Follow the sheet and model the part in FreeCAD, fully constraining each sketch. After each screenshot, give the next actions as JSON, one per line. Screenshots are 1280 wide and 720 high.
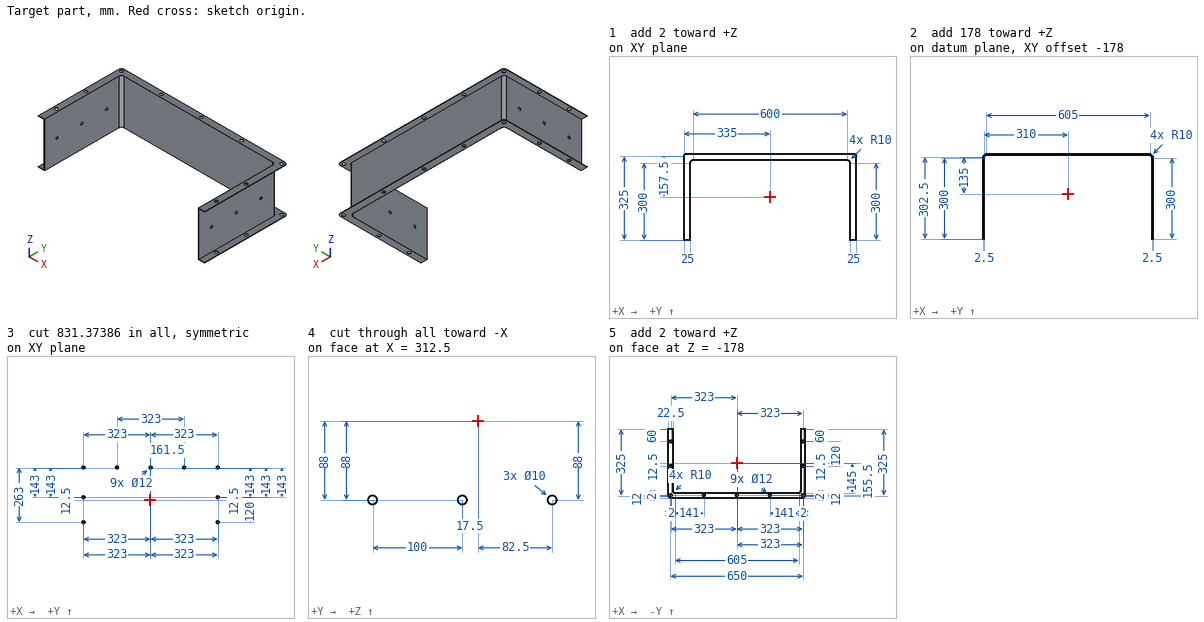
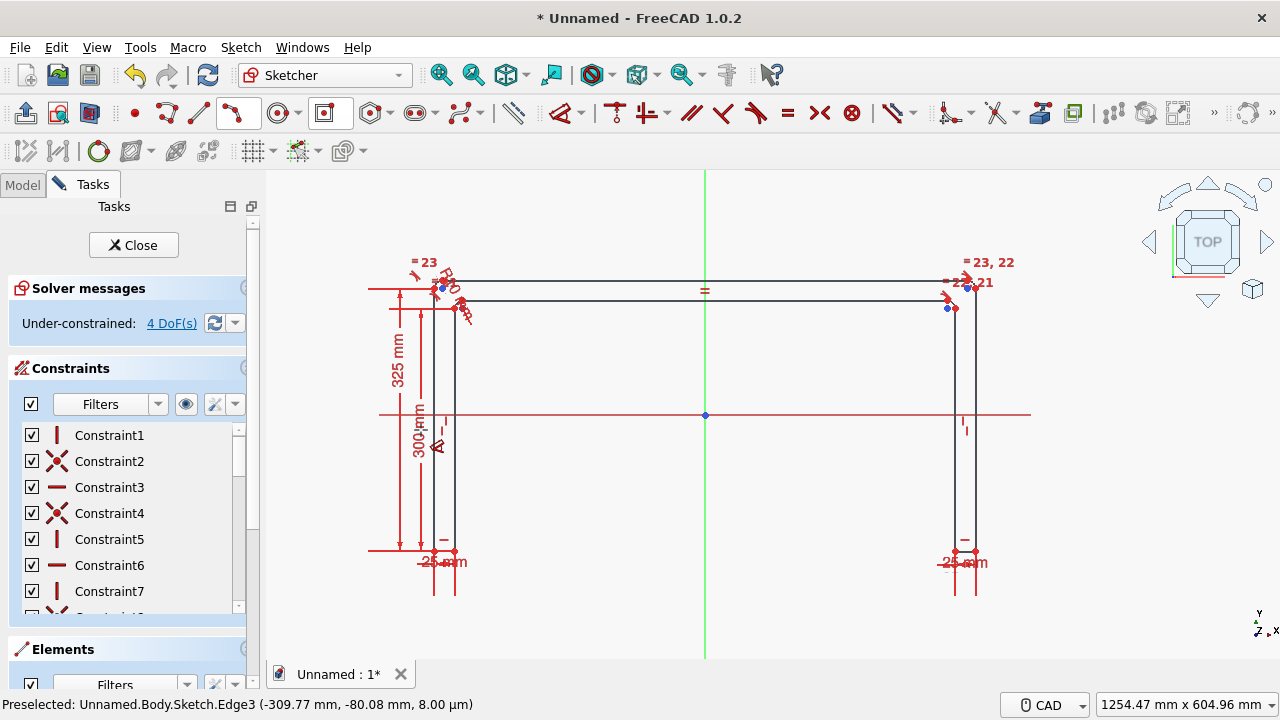
{"action": "left_click", "coordinate": [608, 301]}
{"action": "left_click", "coordinate": [594, 267]}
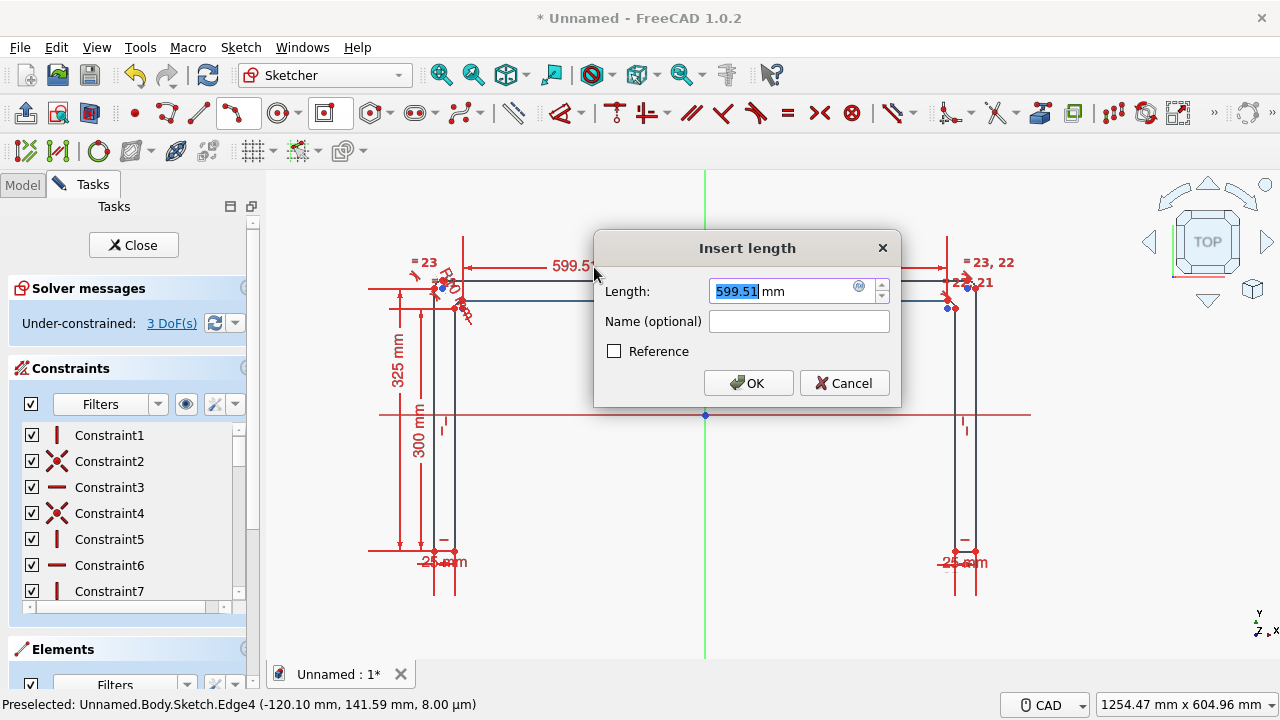
{"action": "type", "text": "600"}
{"action": "key", "text": "Return"}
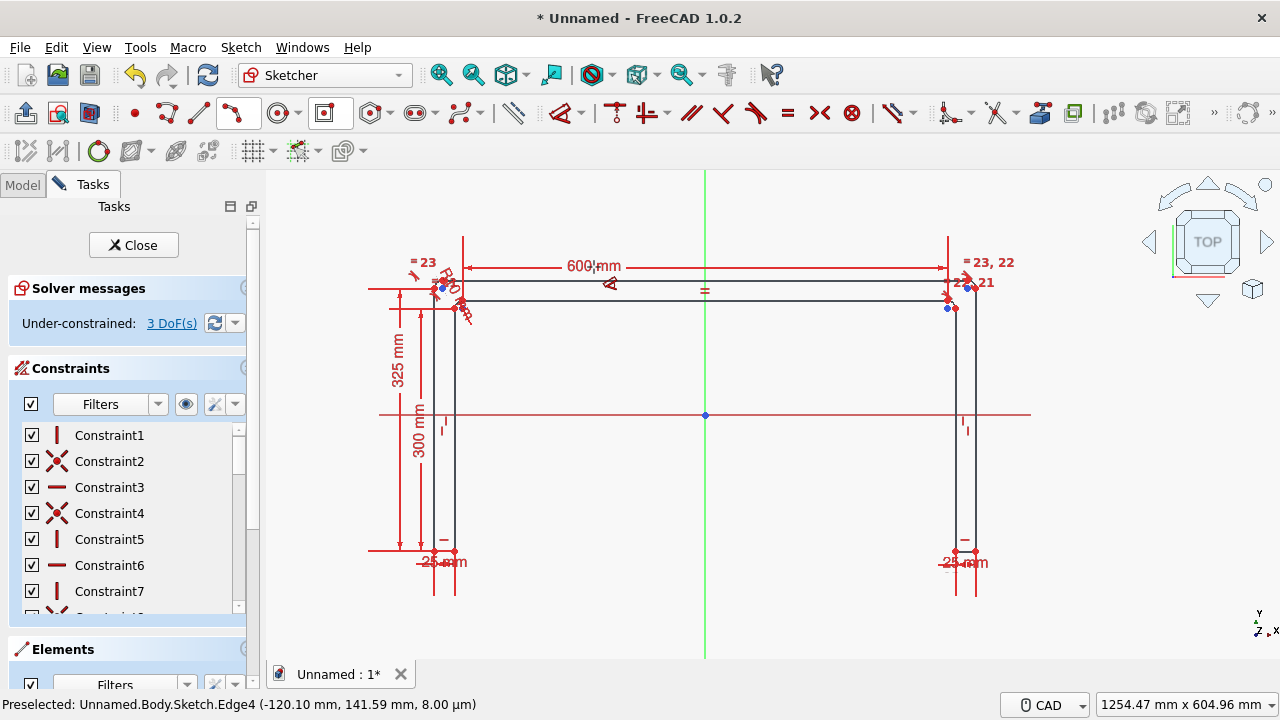
{"action": "left_click", "coordinate": [956, 382]}
{"action": "left_click", "coordinate": [990, 430]}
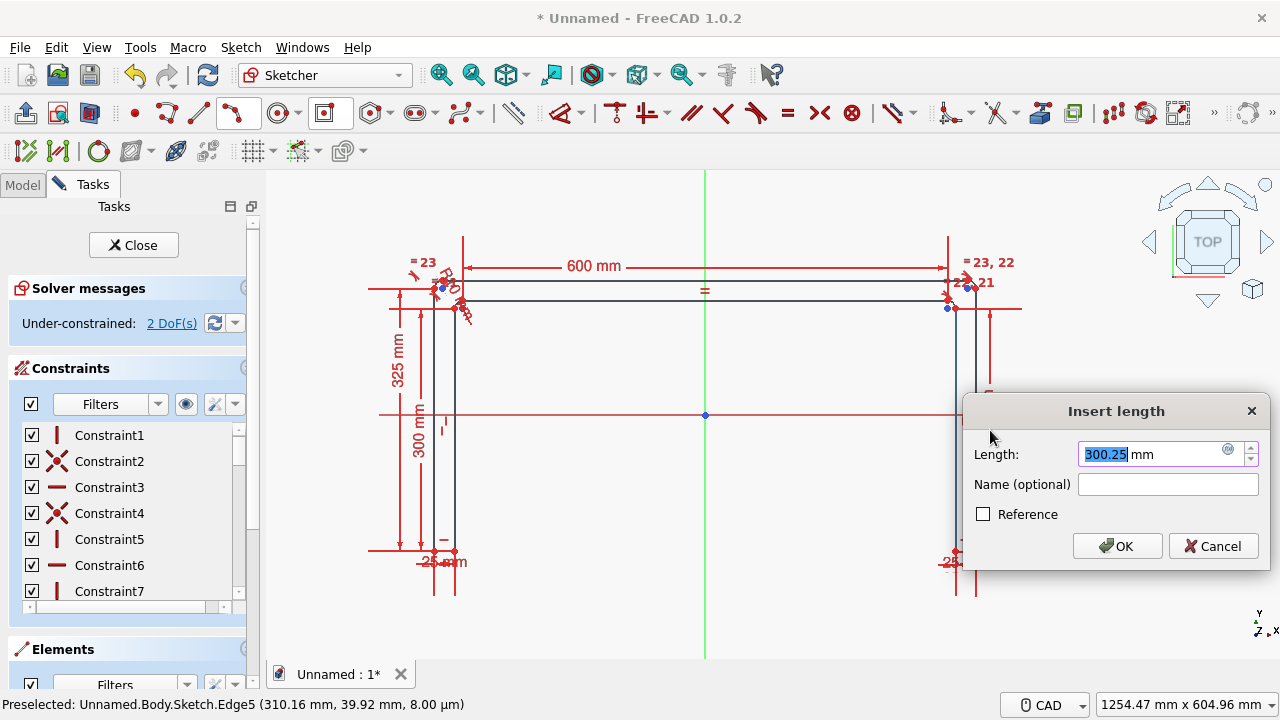
{"action": "type", "text": "300"}
{"action": "key", "text": "Return"}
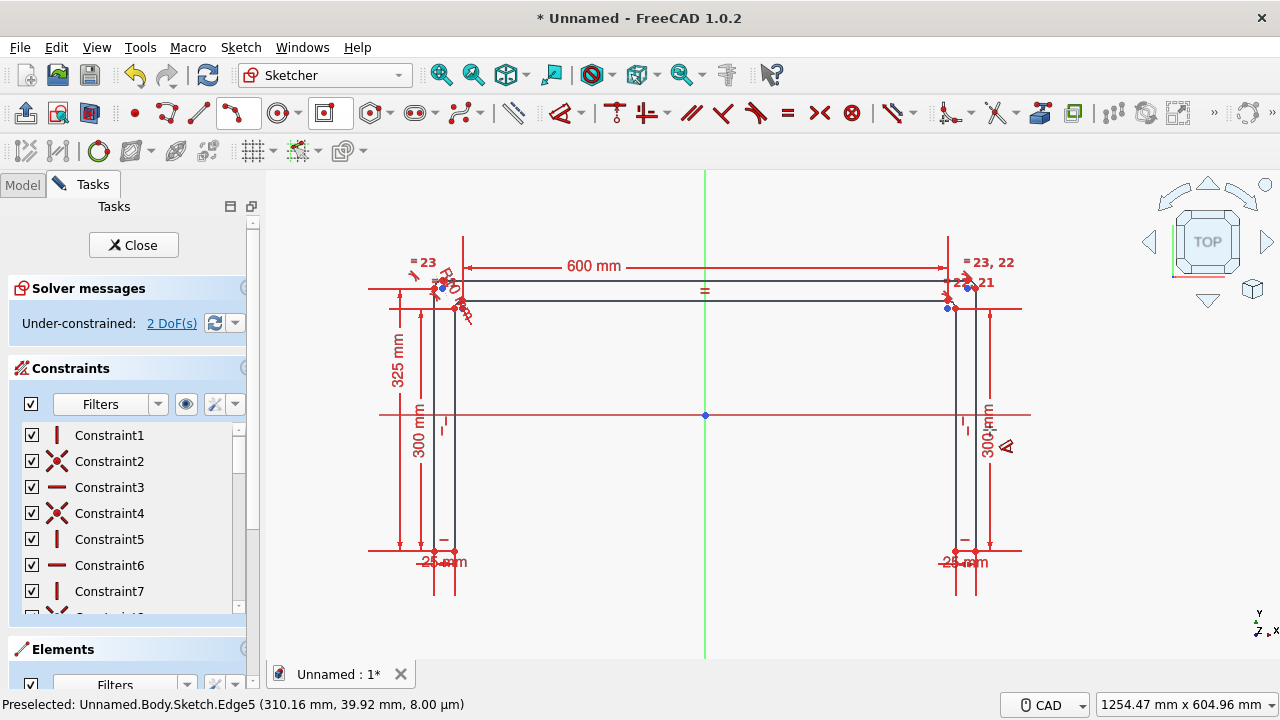
{"action": "scroll", "coordinate": [434, 289], "scroll_direction": "up", "scroll_amount": 3}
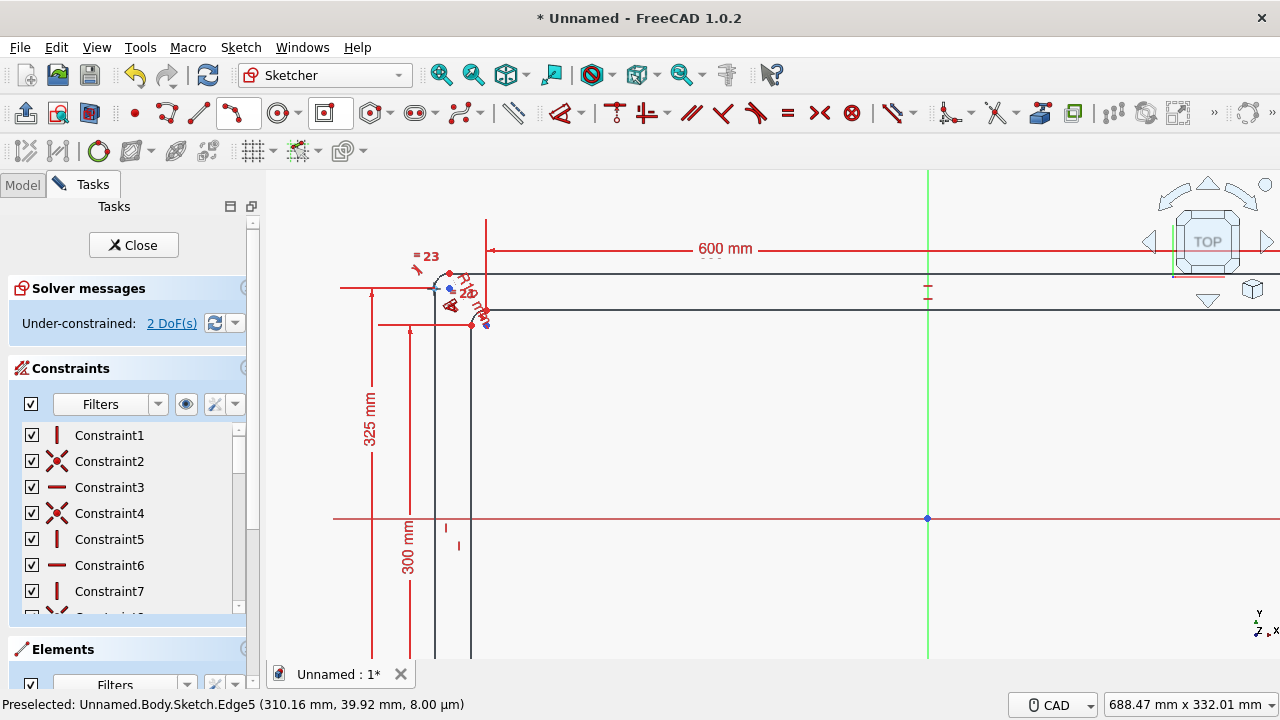
{"action": "left_click", "coordinate": [435, 288]}
{"action": "left_click", "coordinate": [568, 254]}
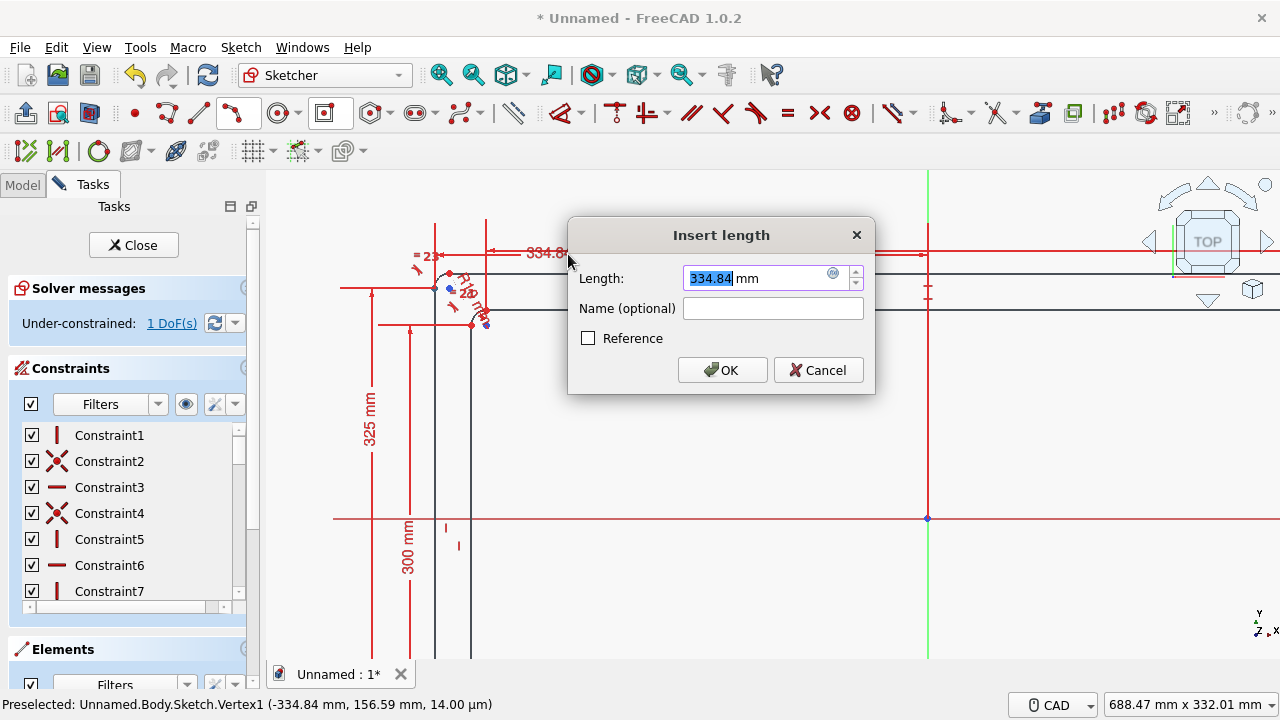
{"action": "type", "text": "335"}
{"action": "key", "text": "Return"}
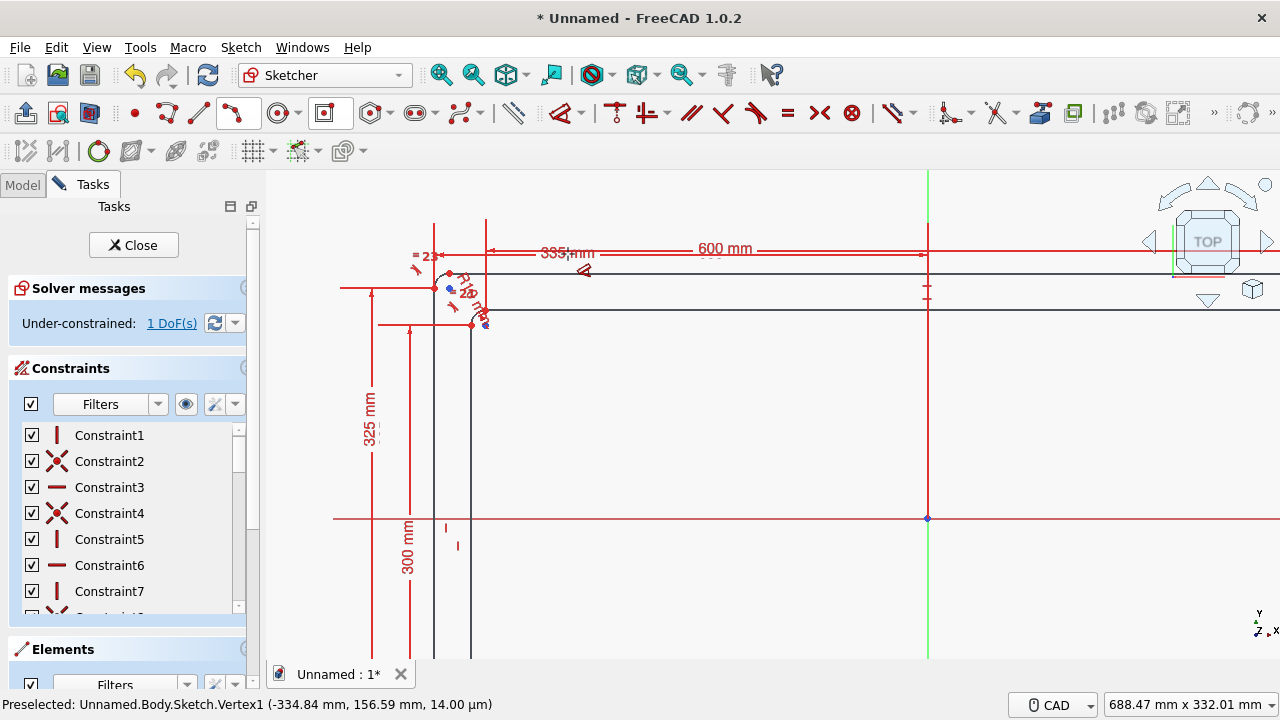
{"action": "left_click", "coordinate": [434, 288]}
{"action": "left_click", "coordinate": [400, 351]}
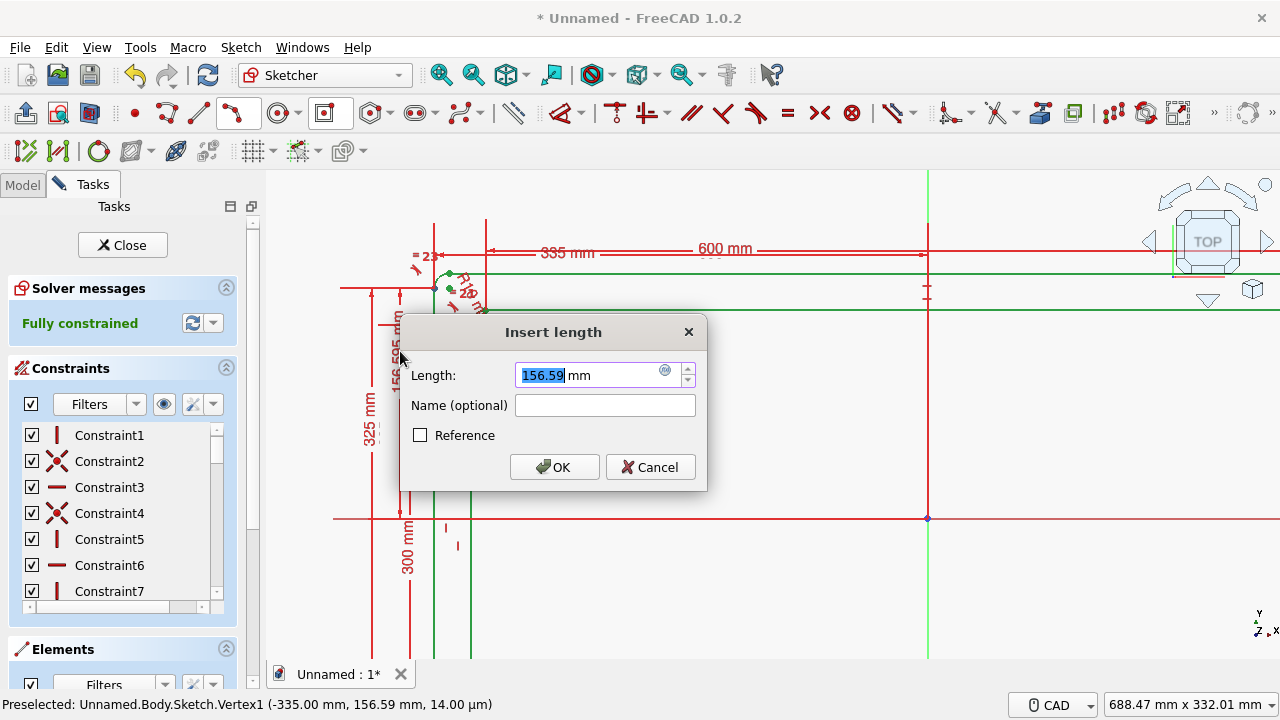
{"action": "type", "text": "157.5"}
{"action": "key", "text": "Return"}
{"action": "key", "text": "Escape"}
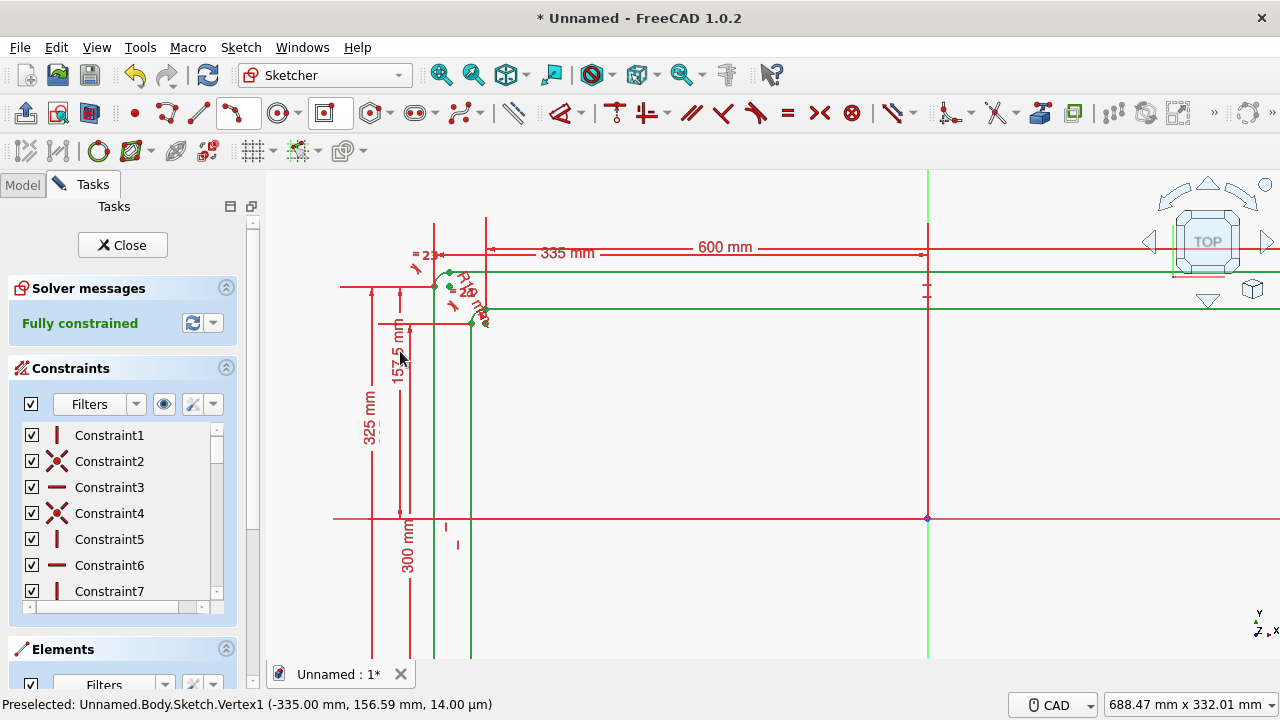
{"action": "left_click", "coordinate": [123, 245]}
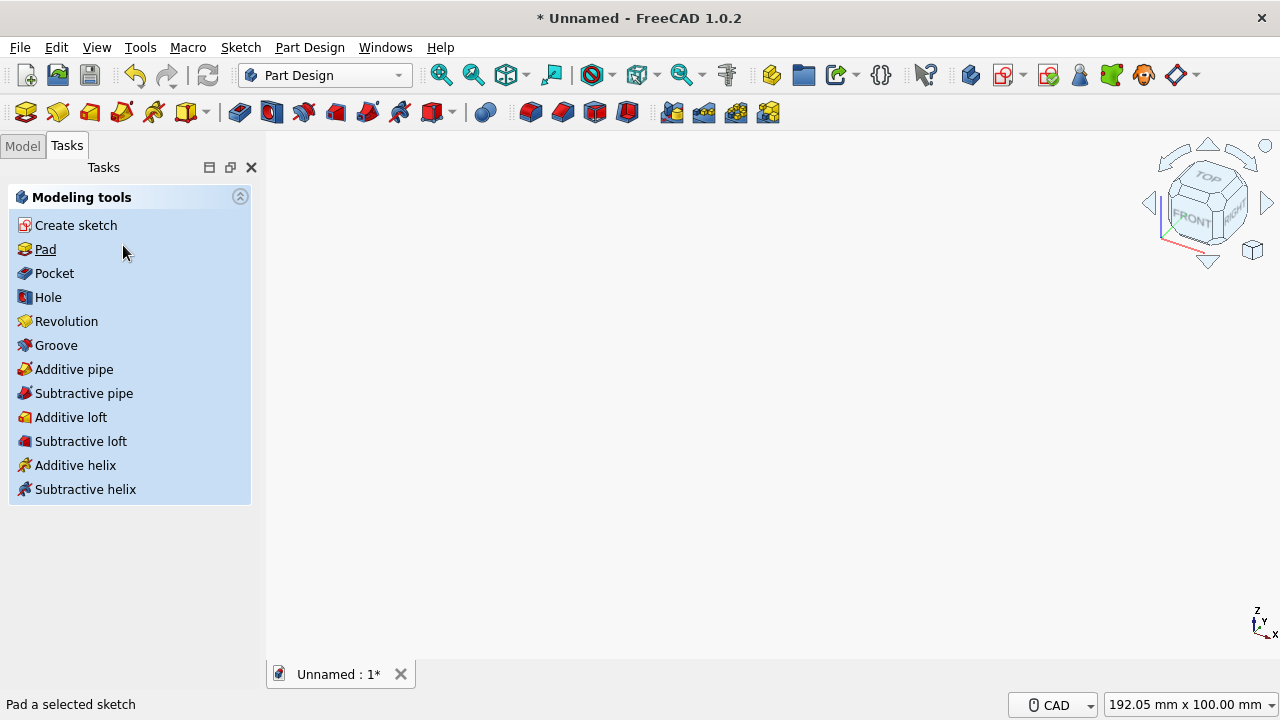
{"action": "left_click", "coordinate": [26, 112]}